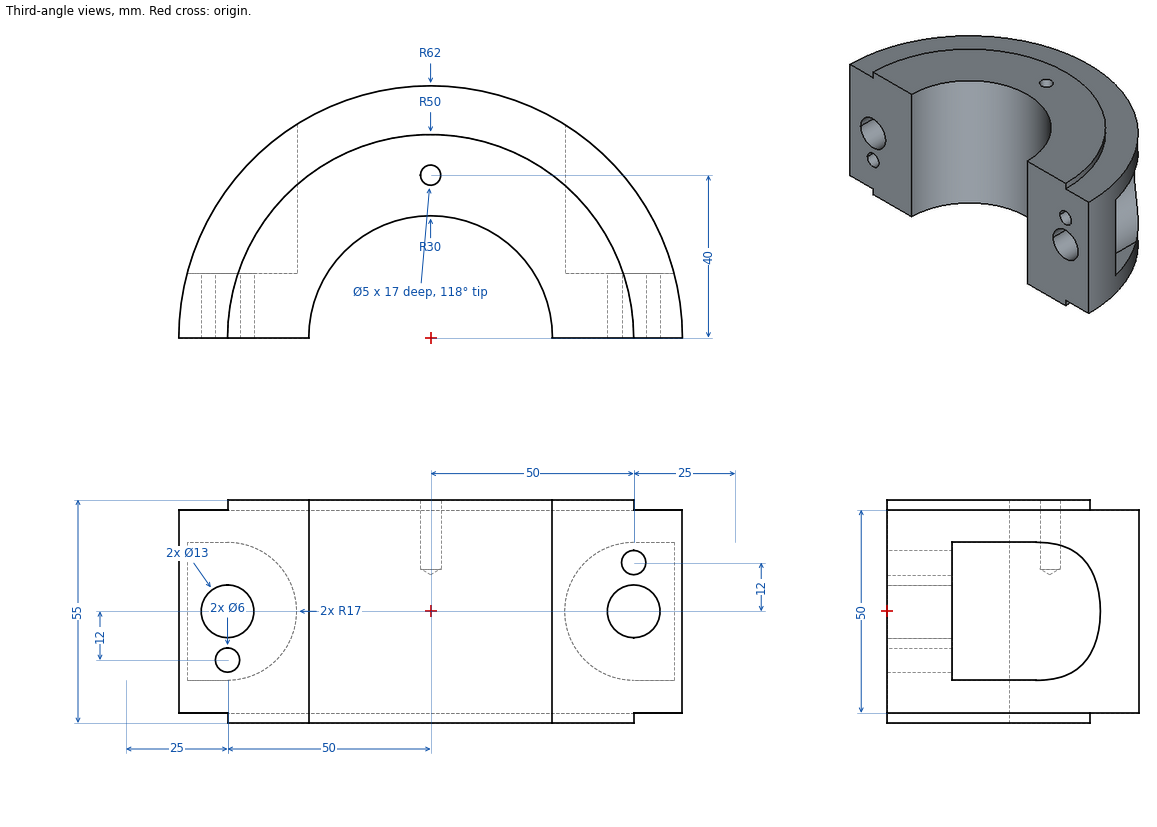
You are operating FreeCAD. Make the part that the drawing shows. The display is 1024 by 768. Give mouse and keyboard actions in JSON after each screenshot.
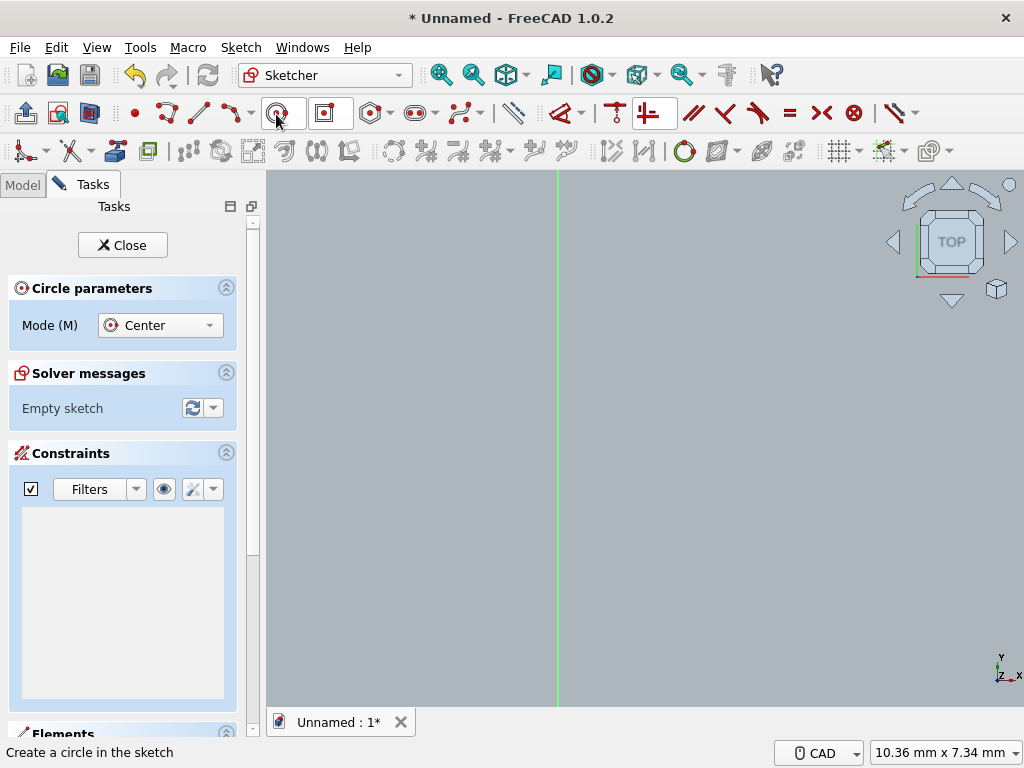
{"action": "left_click", "coordinate": [558, 429]}
{"action": "mouse_move", "coordinate": [687, 299]}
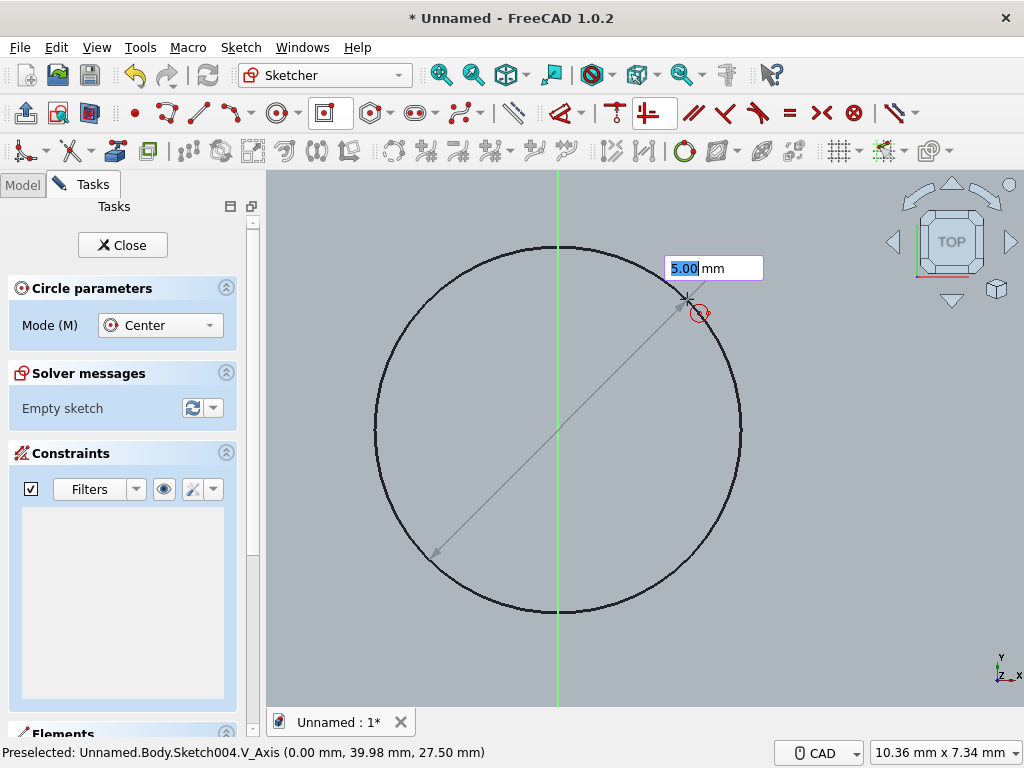
{"action": "type", "text": "5"}
{"action": "key", "text": "Return"}
{"action": "key", "text": "Escape"}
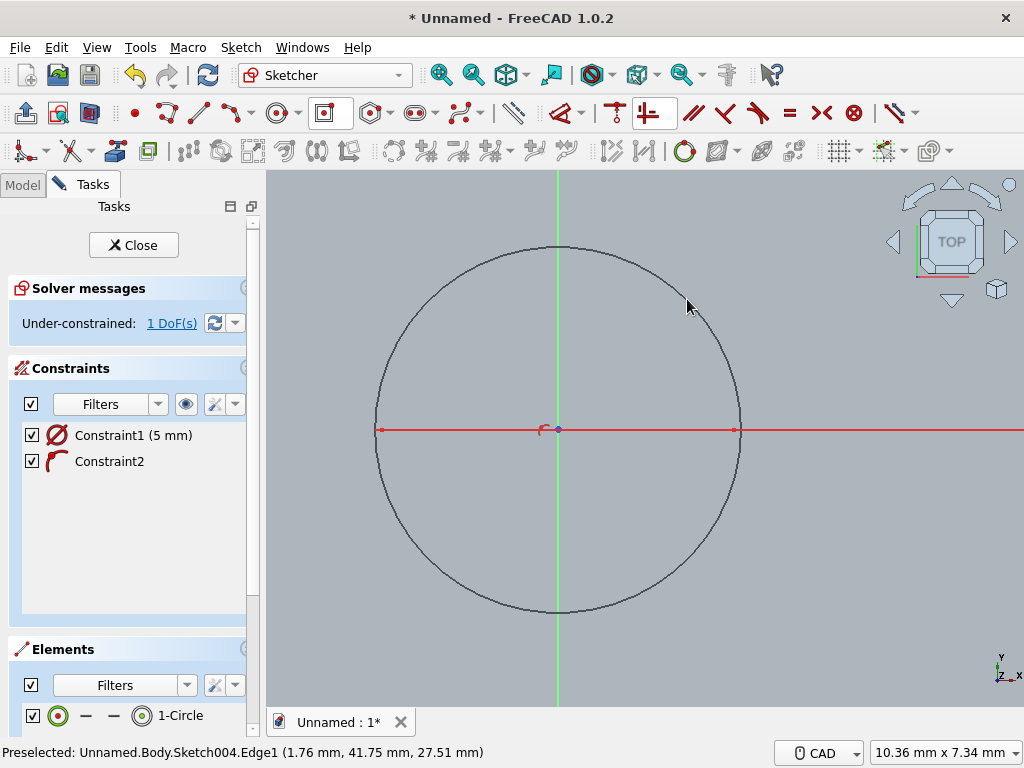
{"action": "left_click", "coordinate": [560, 114]}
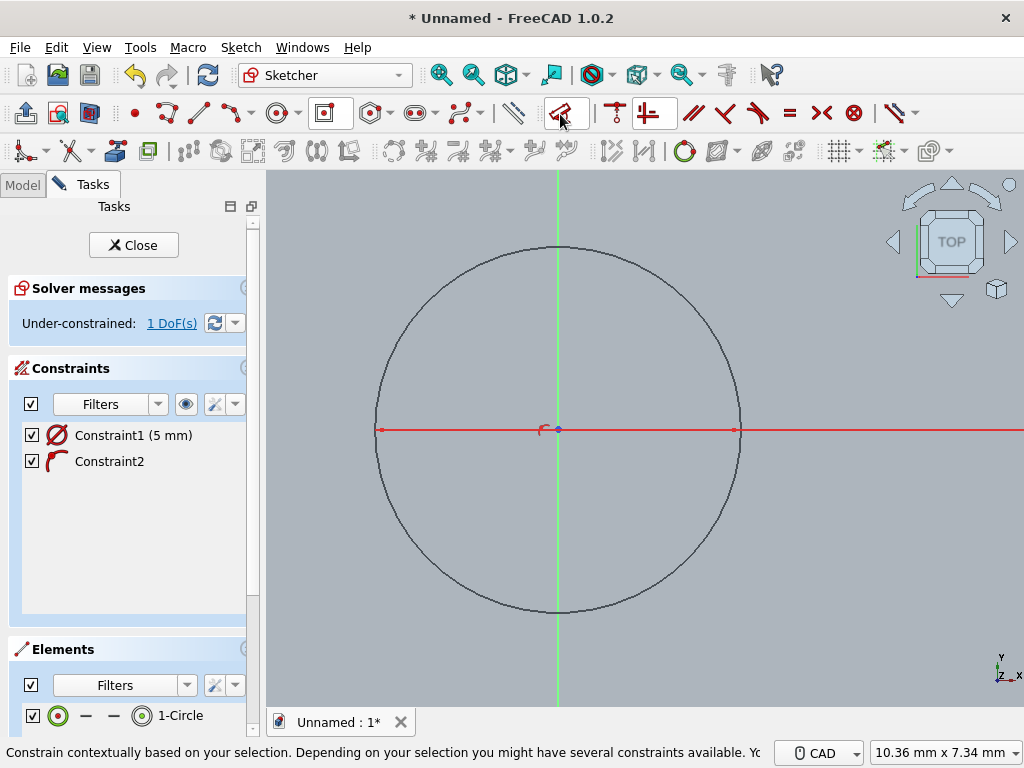
{"action": "left_click", "coordinate": [558, 430]}
{"action": "left_click", "coordinate": [592, 555]}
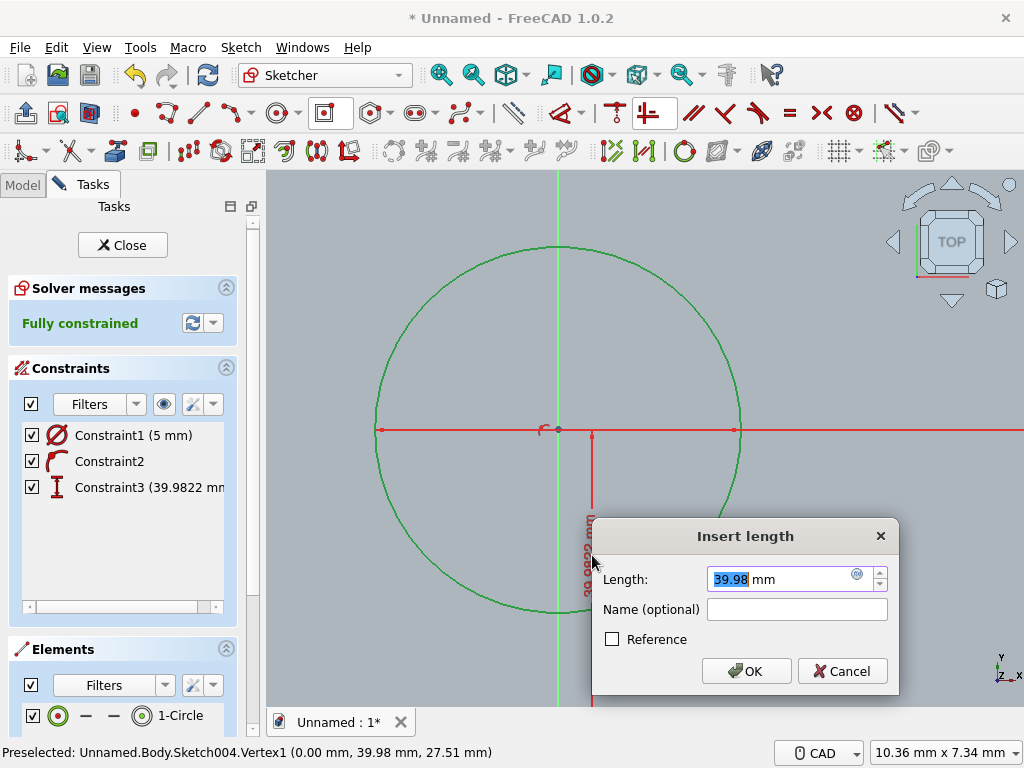
{"action": "type", "text": "40"}
{"action": "key", "text": "Return"}
{"action": "key", "text": "Escape"}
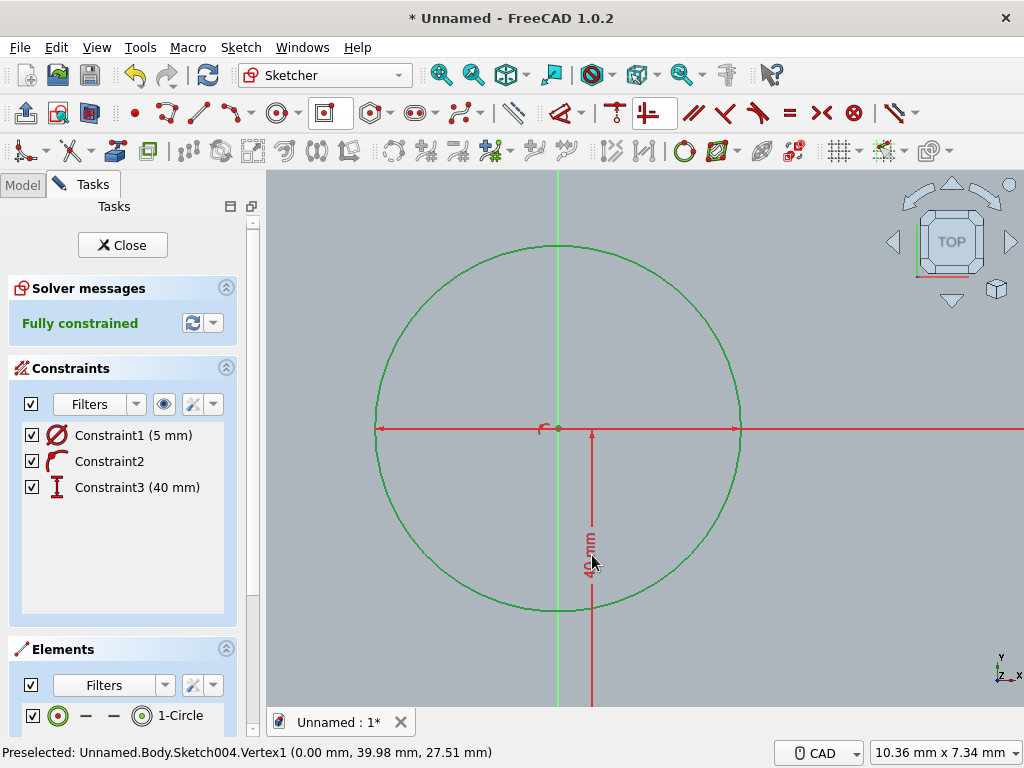
{"action": "left_click", "coordinate": [123, 245]}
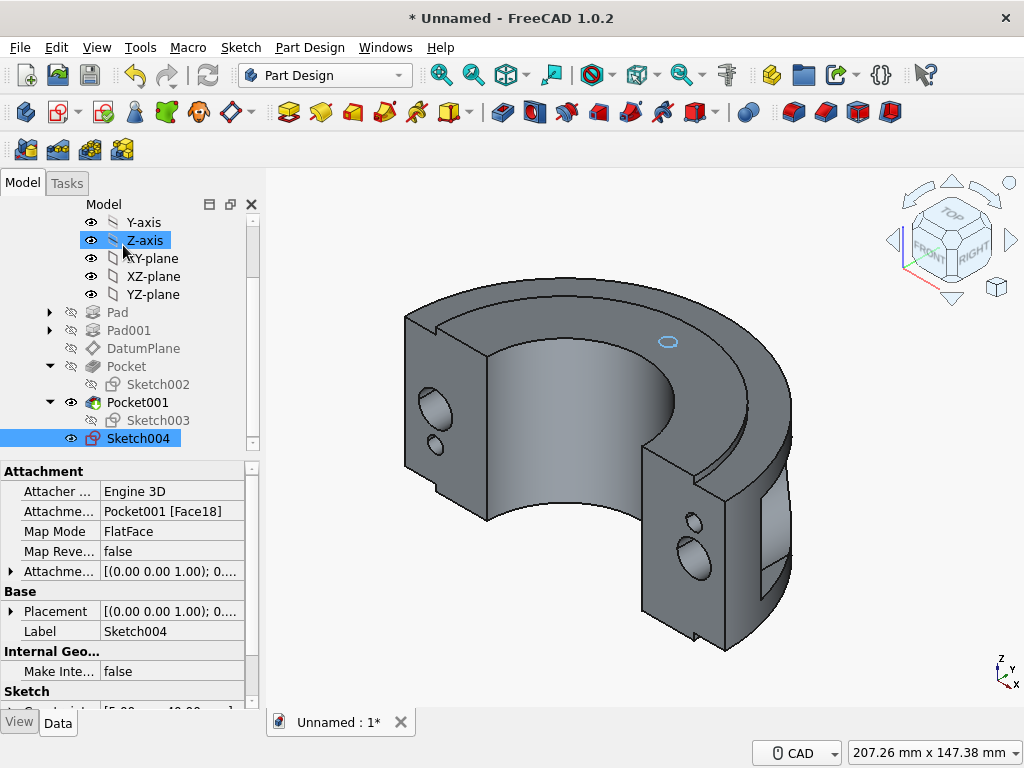
{"action": "left_click", "coordinate": [536, 112]}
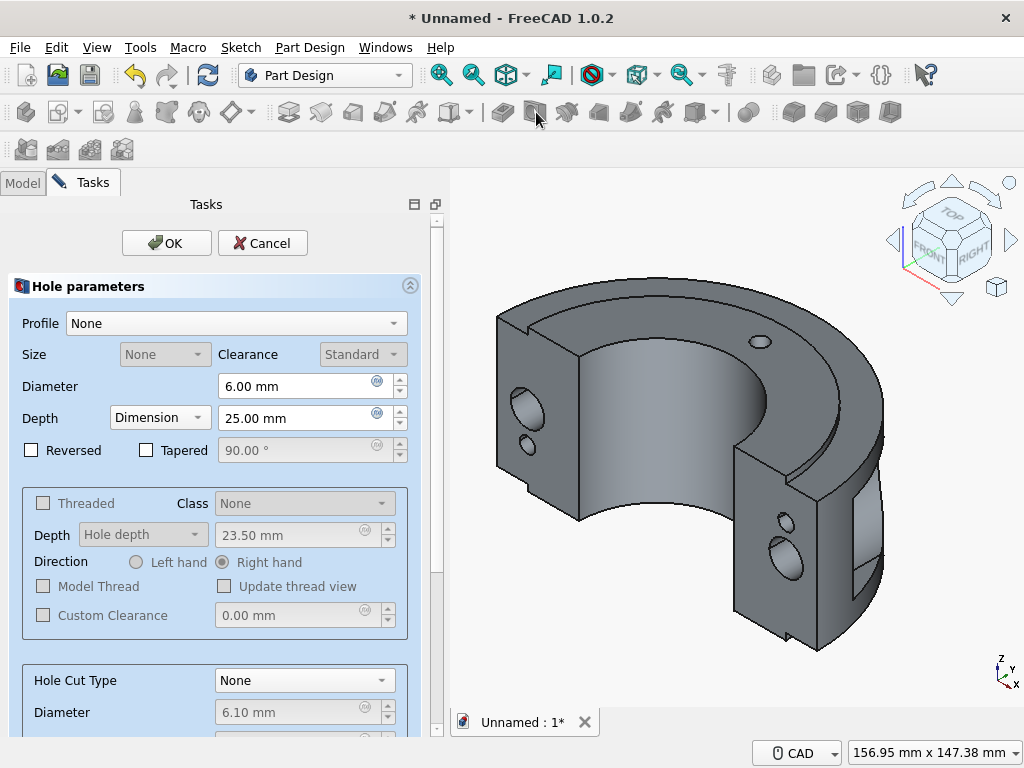
{"action": "triple_click", "coordinate": [305, 386]}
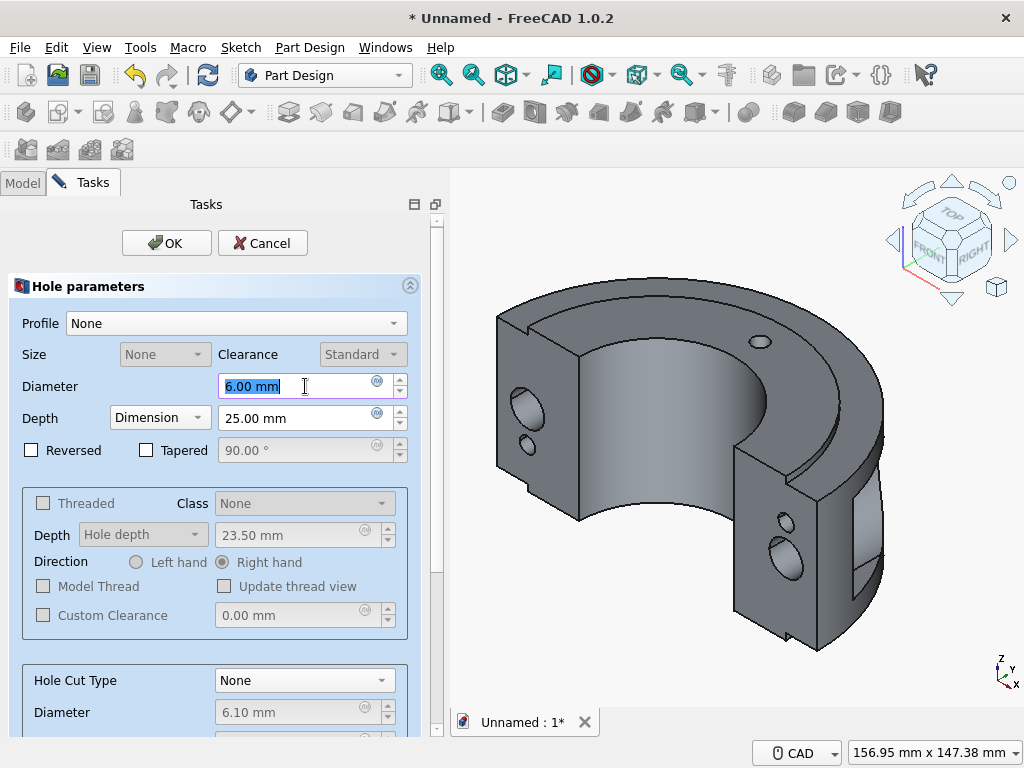
{"action": "type", "text": "5"}
{"action": "key", "text": "Tab"}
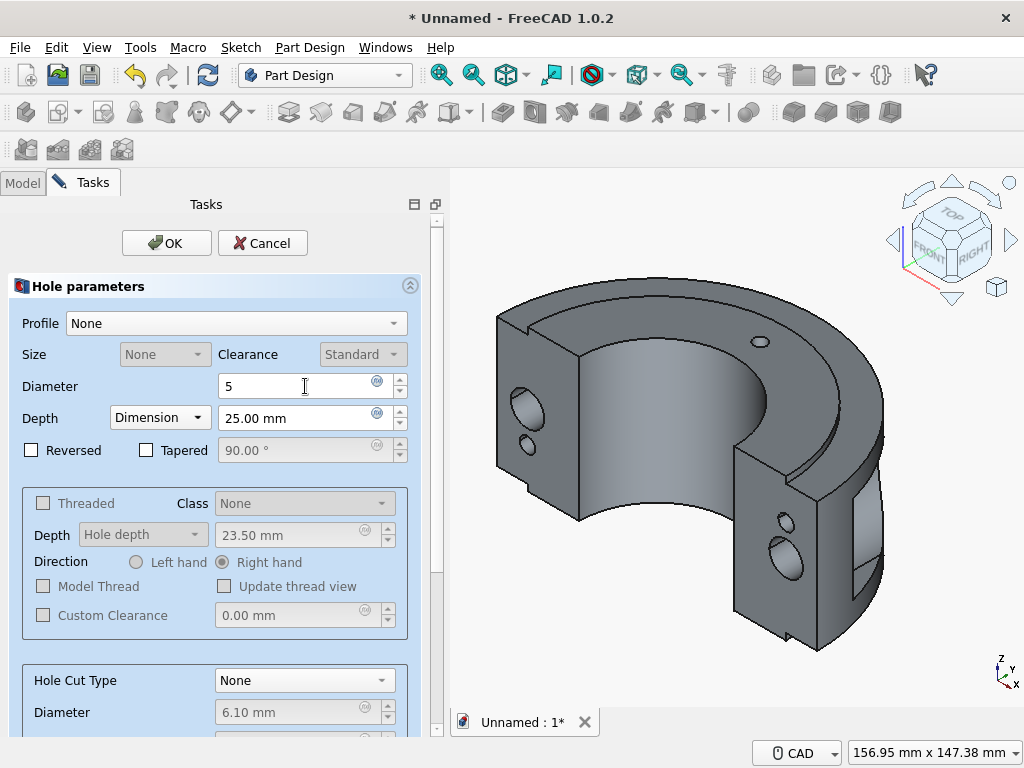
{"action": "triple_click", "coordinate": [305, 418]}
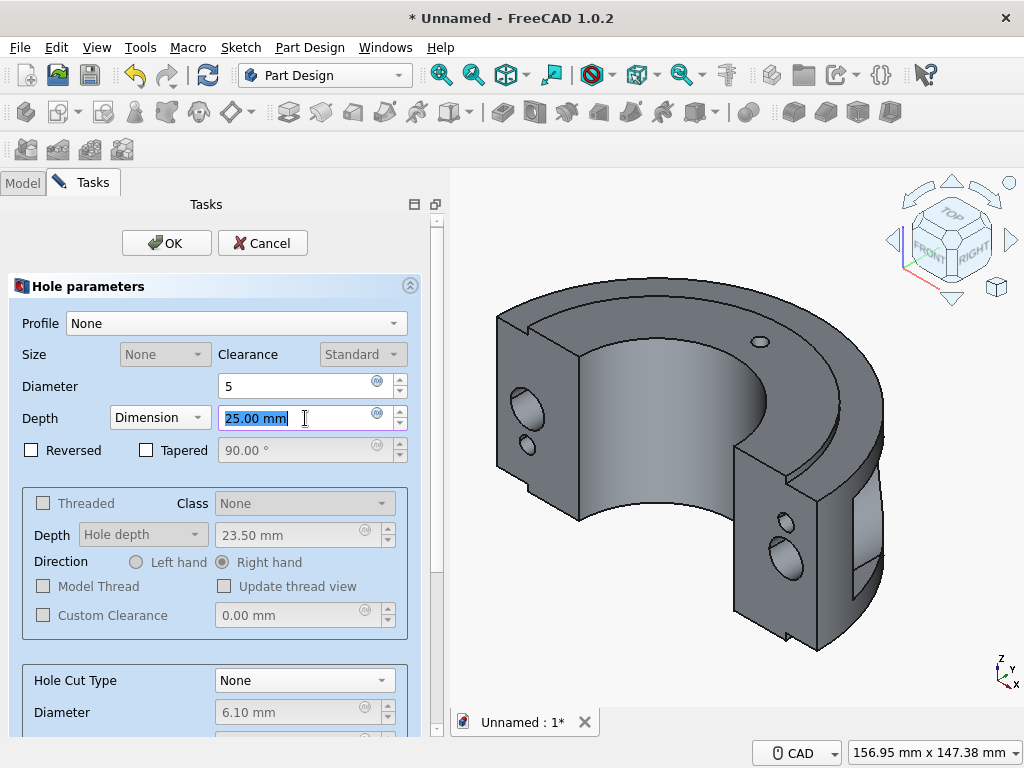
{"action": "type", "text": "17"}
{"action": "key", "text": "Tab"}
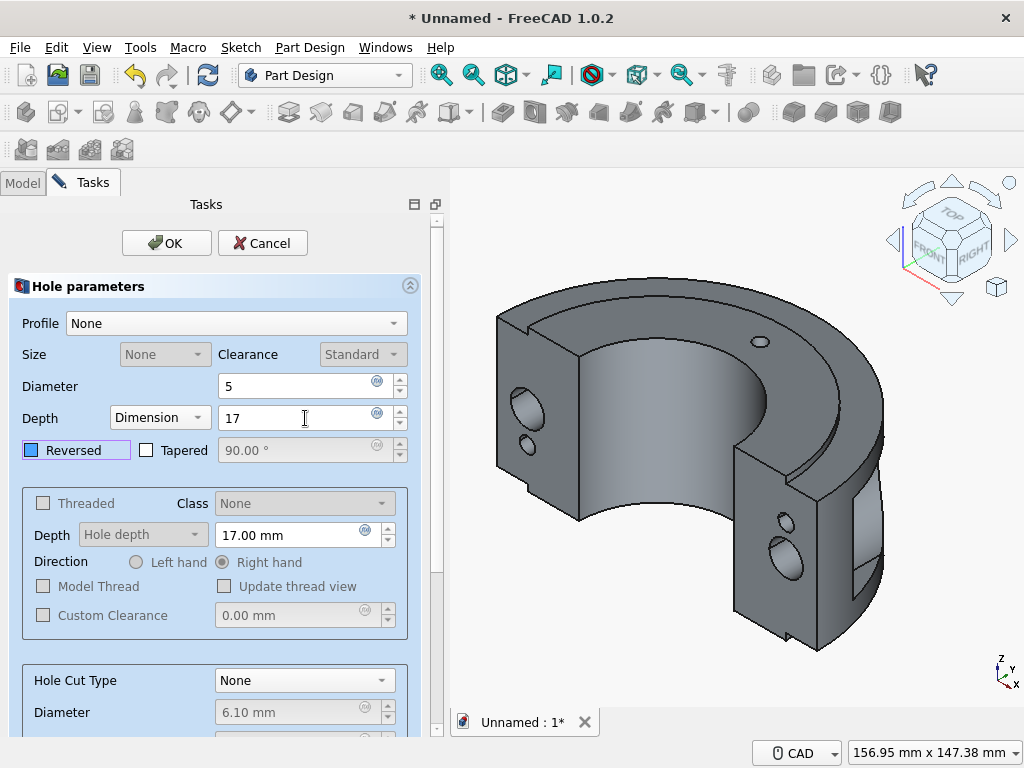
{"action": "left_click", "coordinate": [167, 243]}